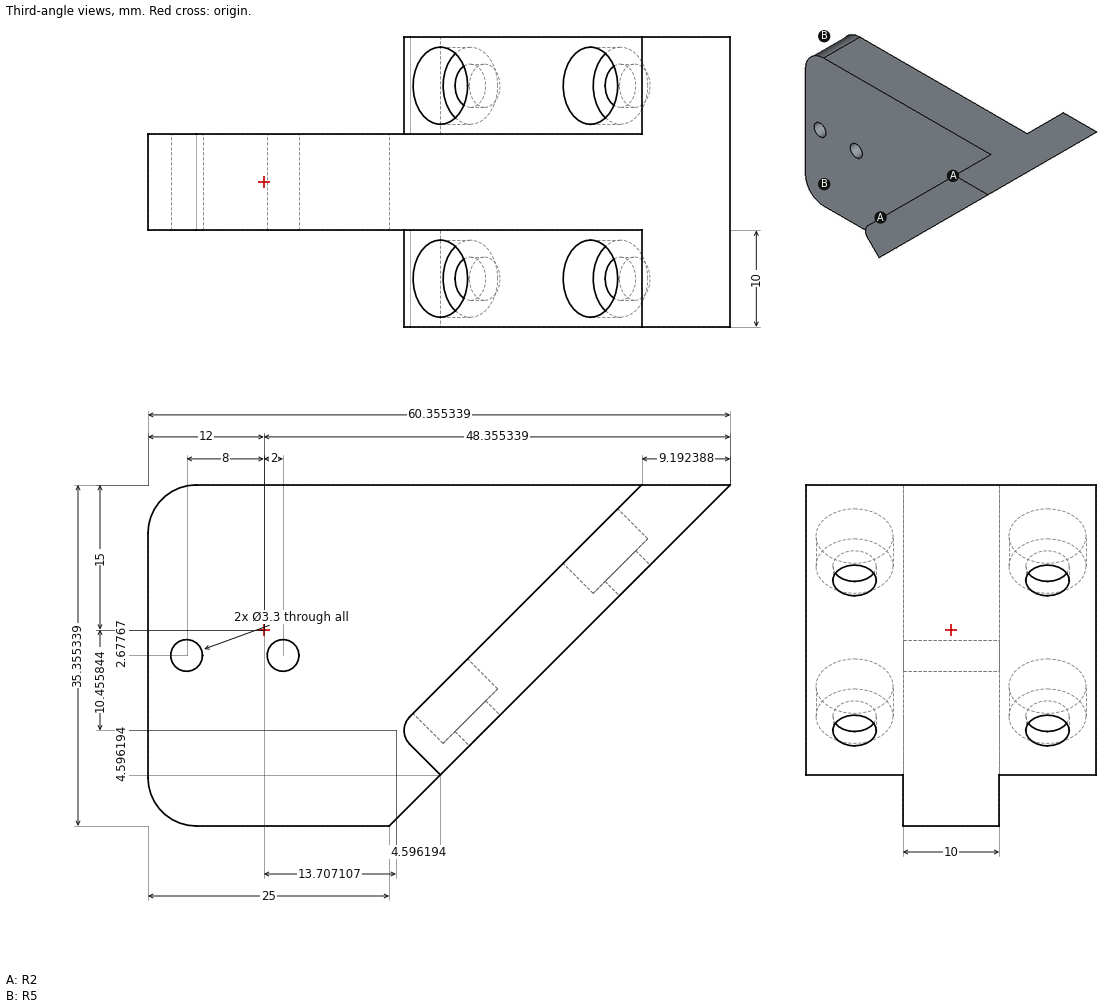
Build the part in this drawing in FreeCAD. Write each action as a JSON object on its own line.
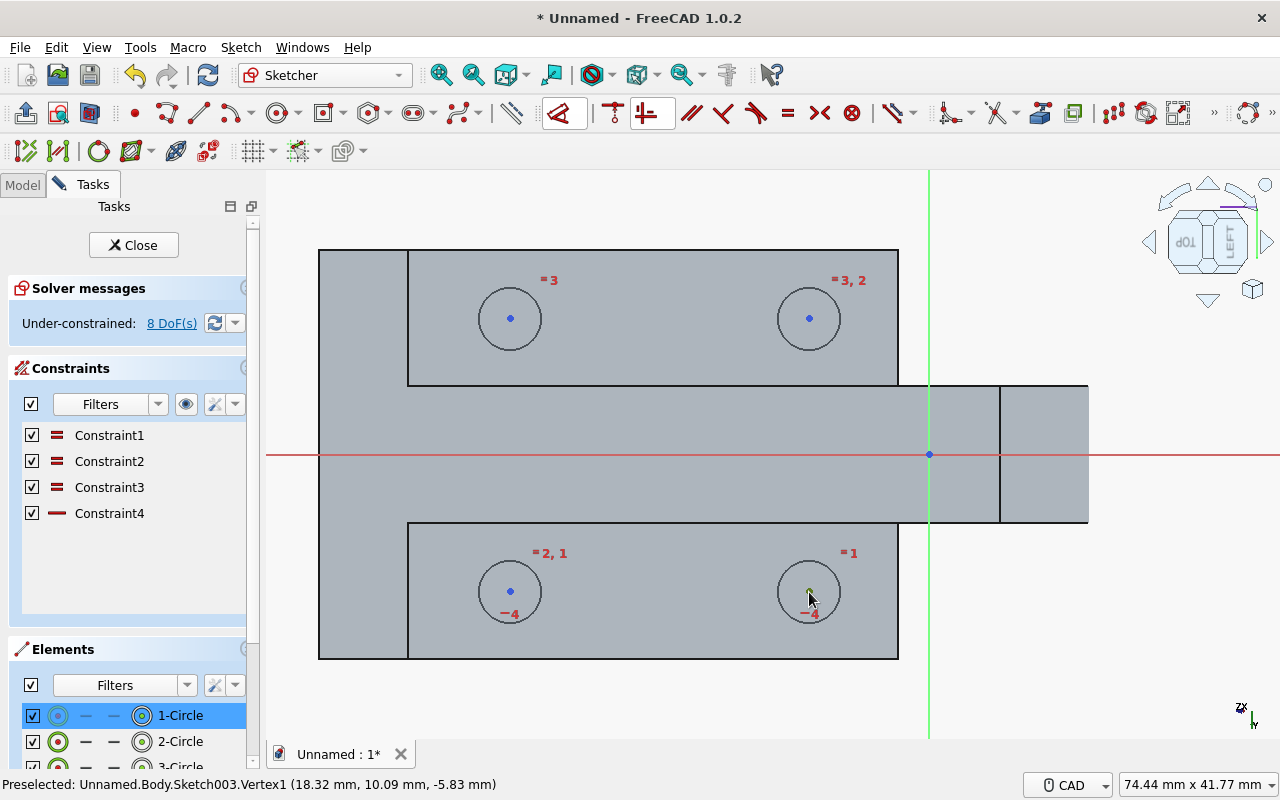
{"action": "left_click", "coordinate": [809, 319]}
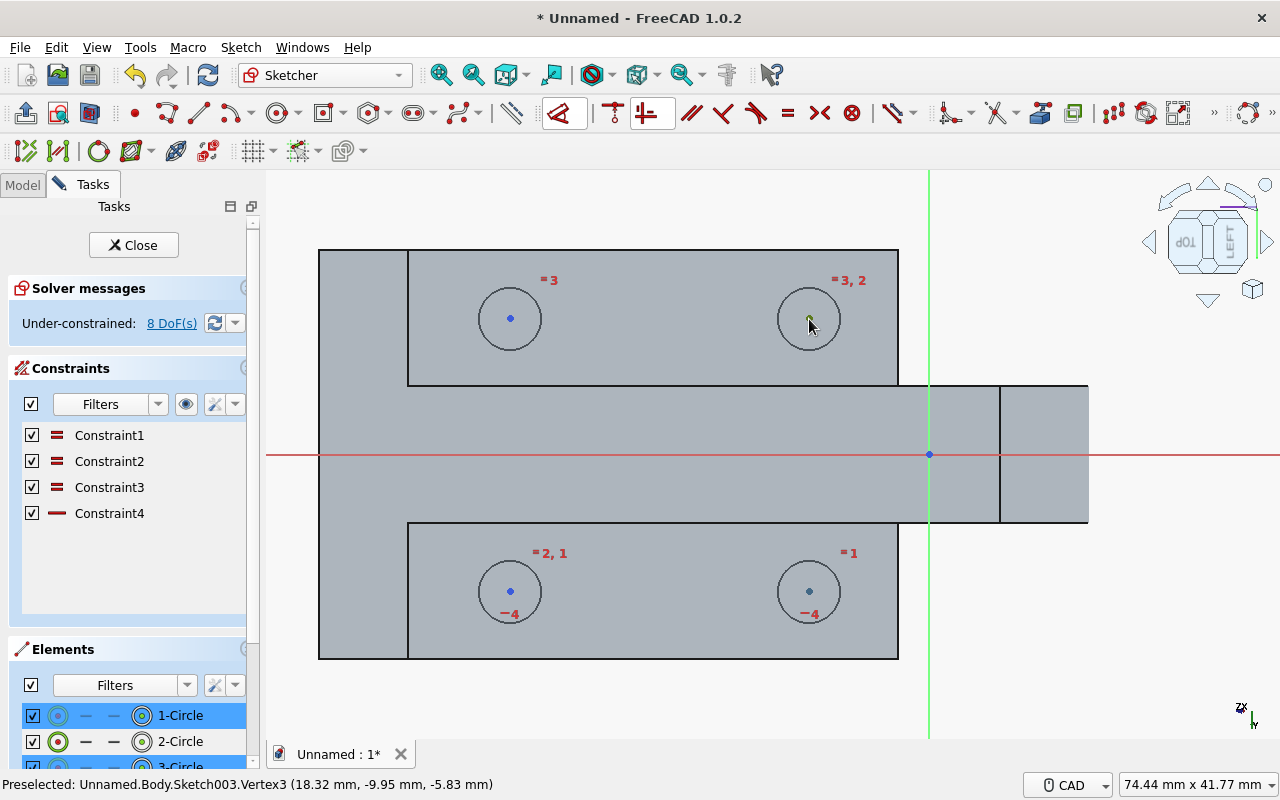
{"action": "left_click", "coordinate": [670, 114]}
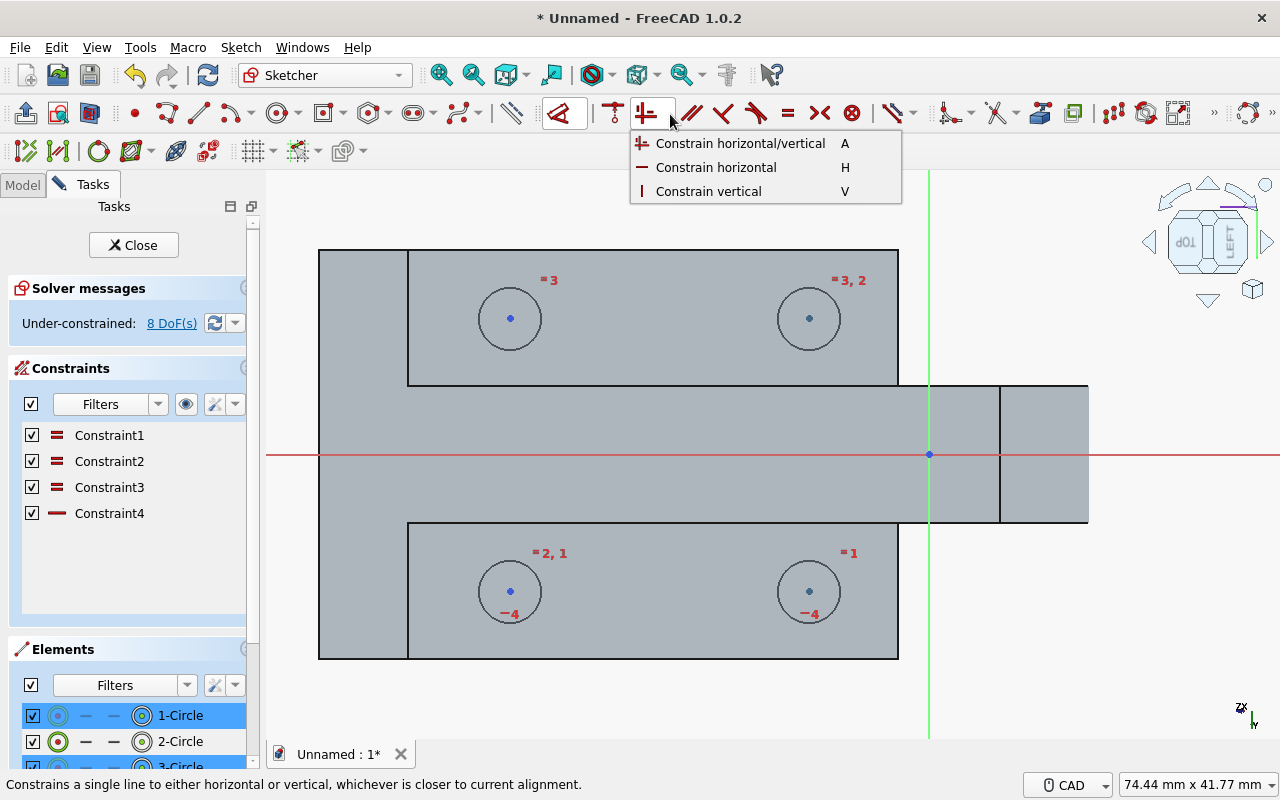
{"action": "left_click", "coordinate": [766, 191]}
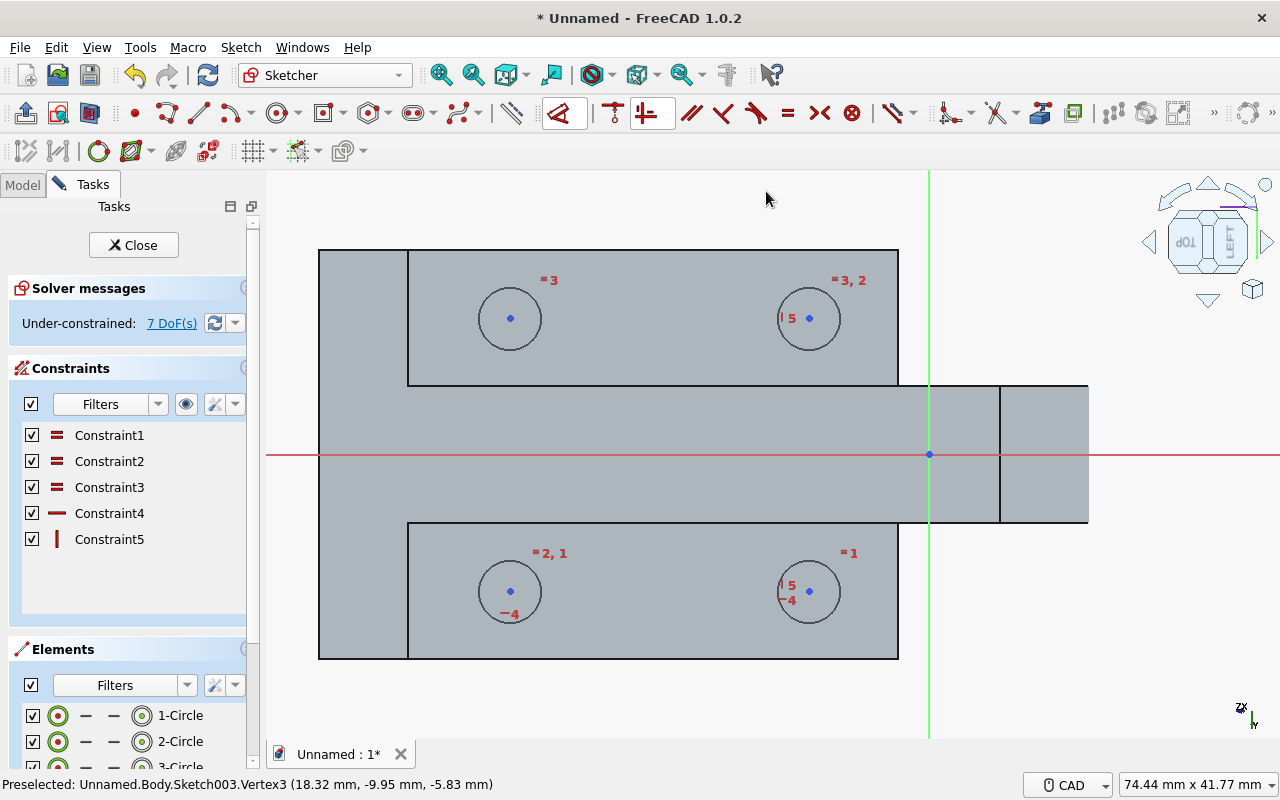
{"action": "left_click", "coordinate": [510, 592]}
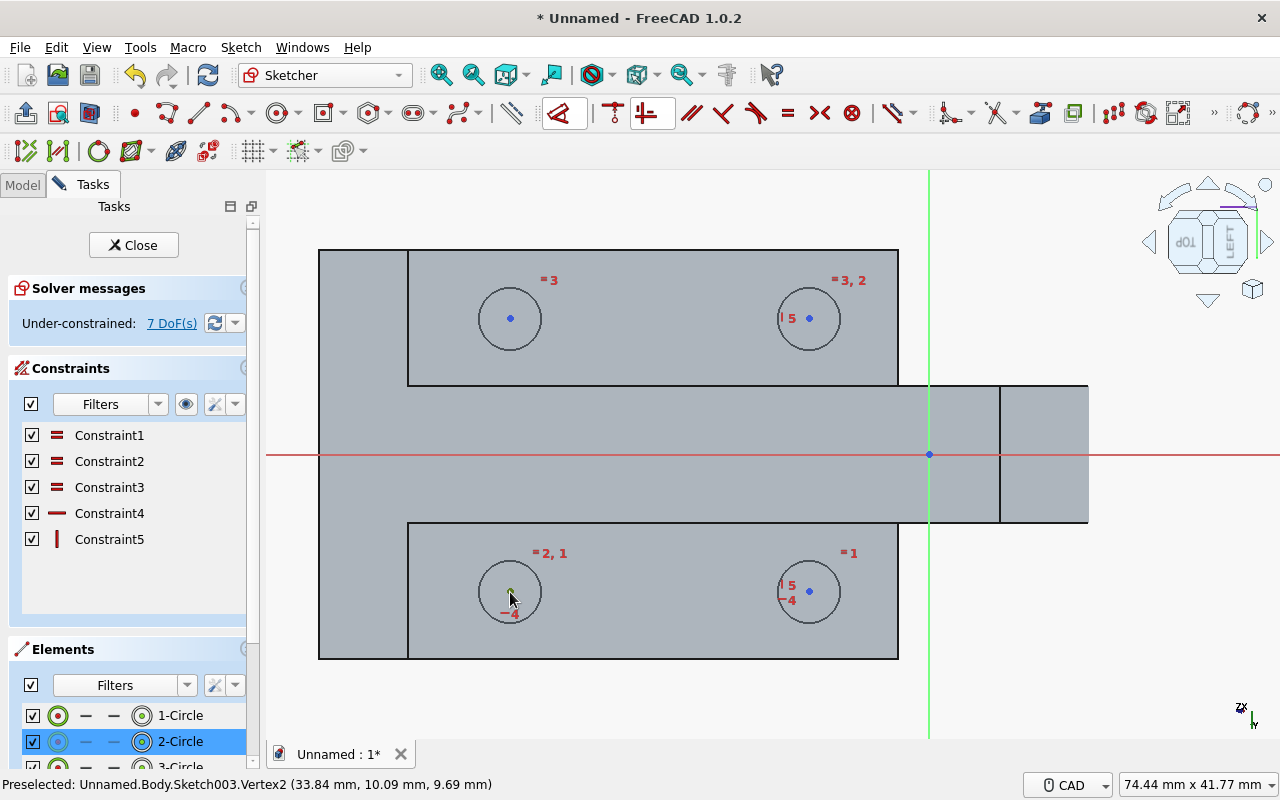
{"action": "left_click", "coordinate": [510, 319]}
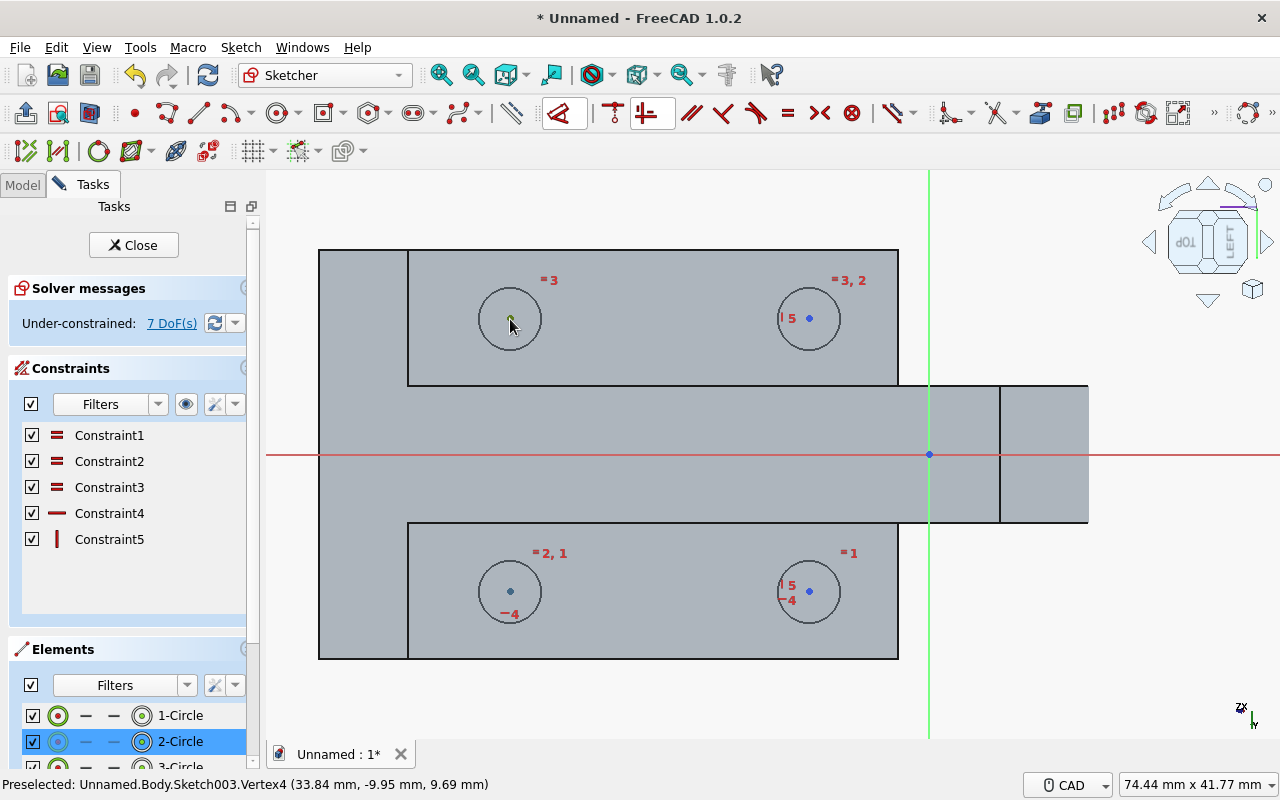
{"action": "left_click", "coordinate": [670, 114]}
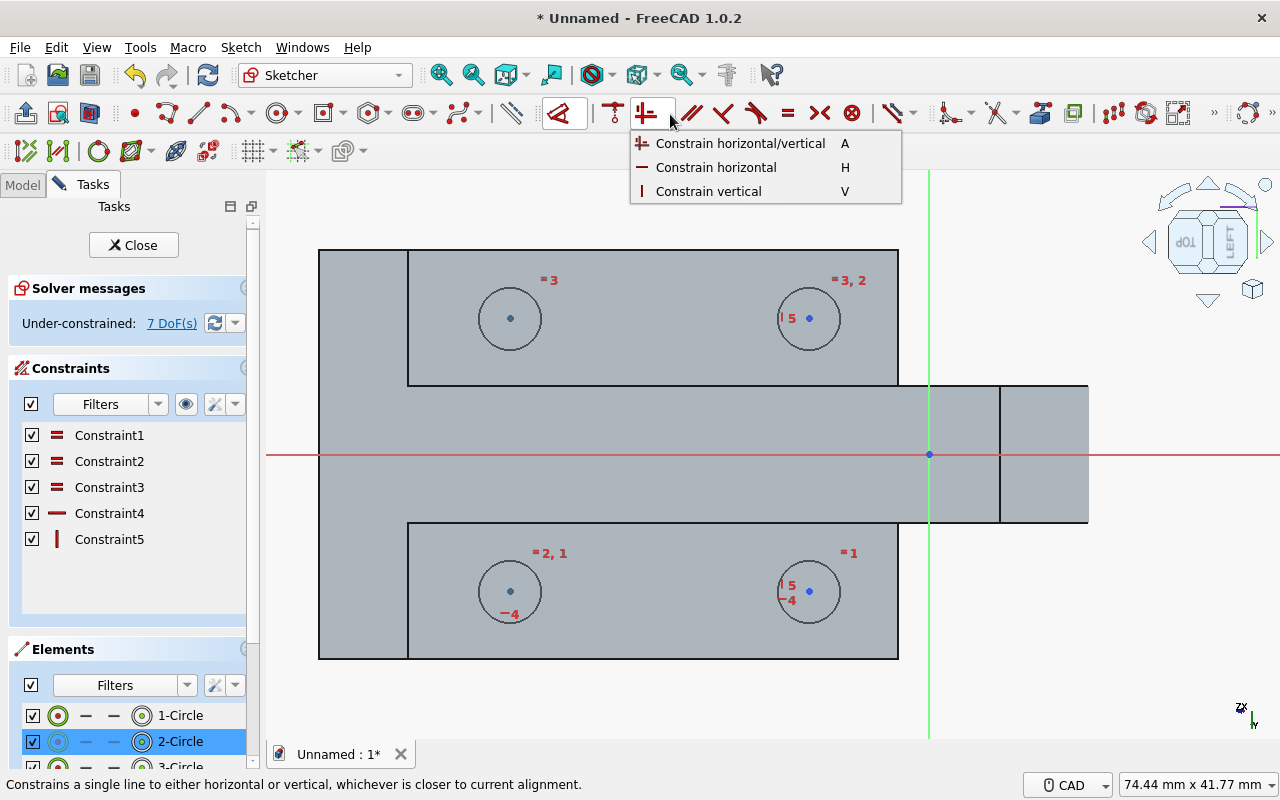
{"action": "left_click", "coordinate": [766, 191]}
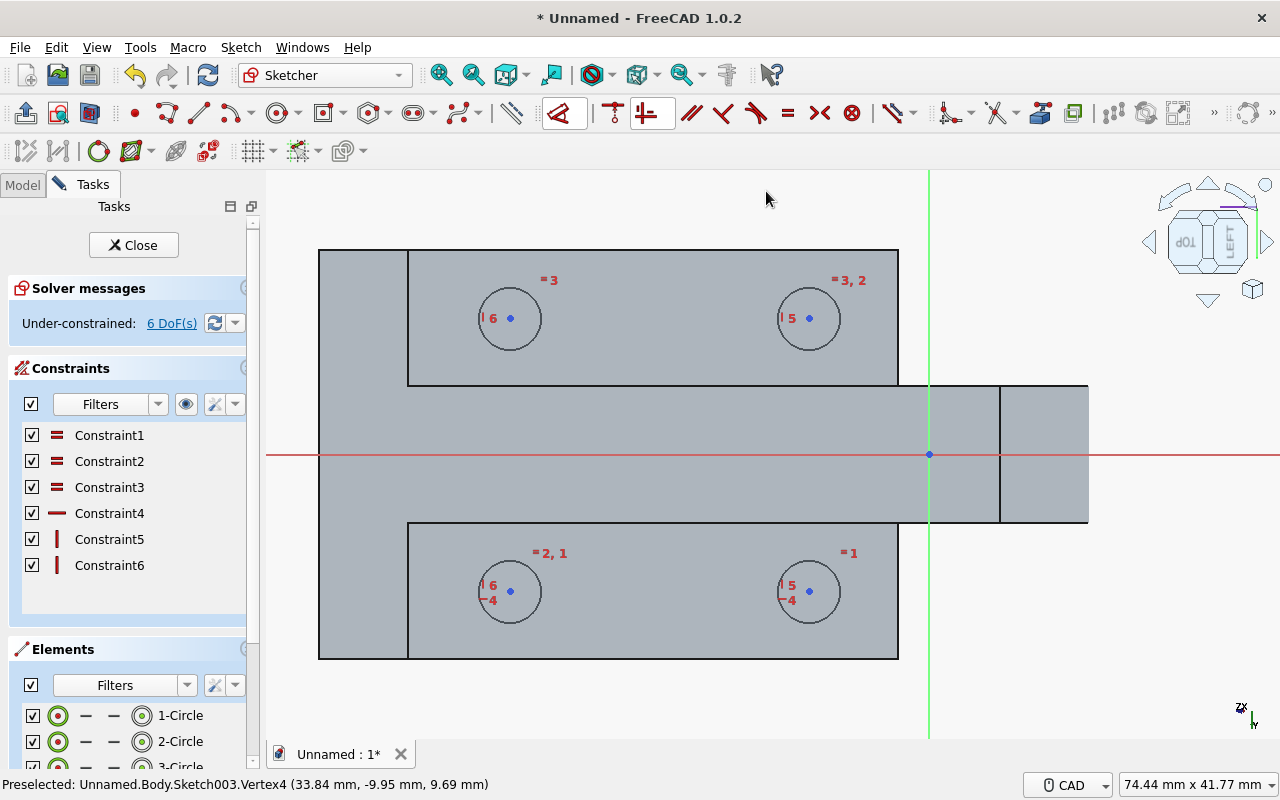
{"action": "left_click", "coordinate": [809, 319]}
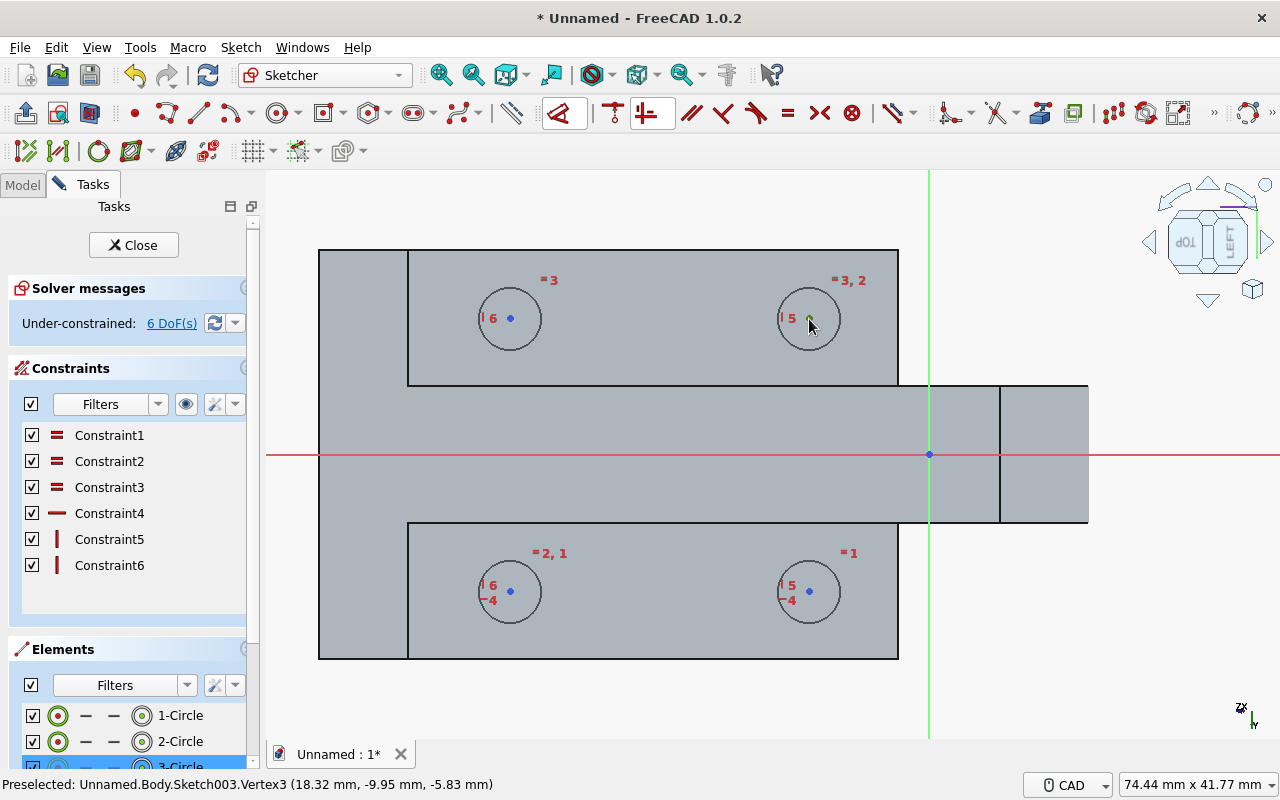
{"action": "left_click", "coordinate": [510, 319]}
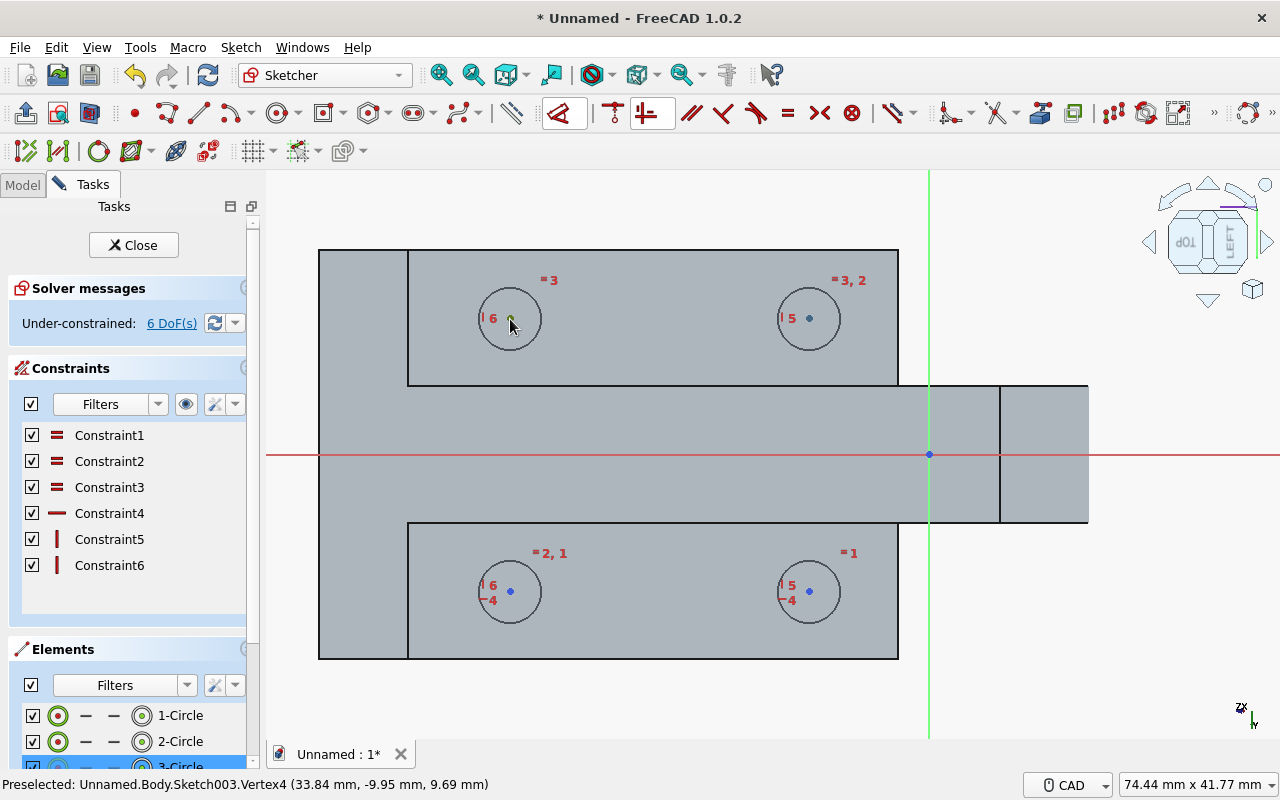
{"action": "left_click", "coordinate": [670, 114]}